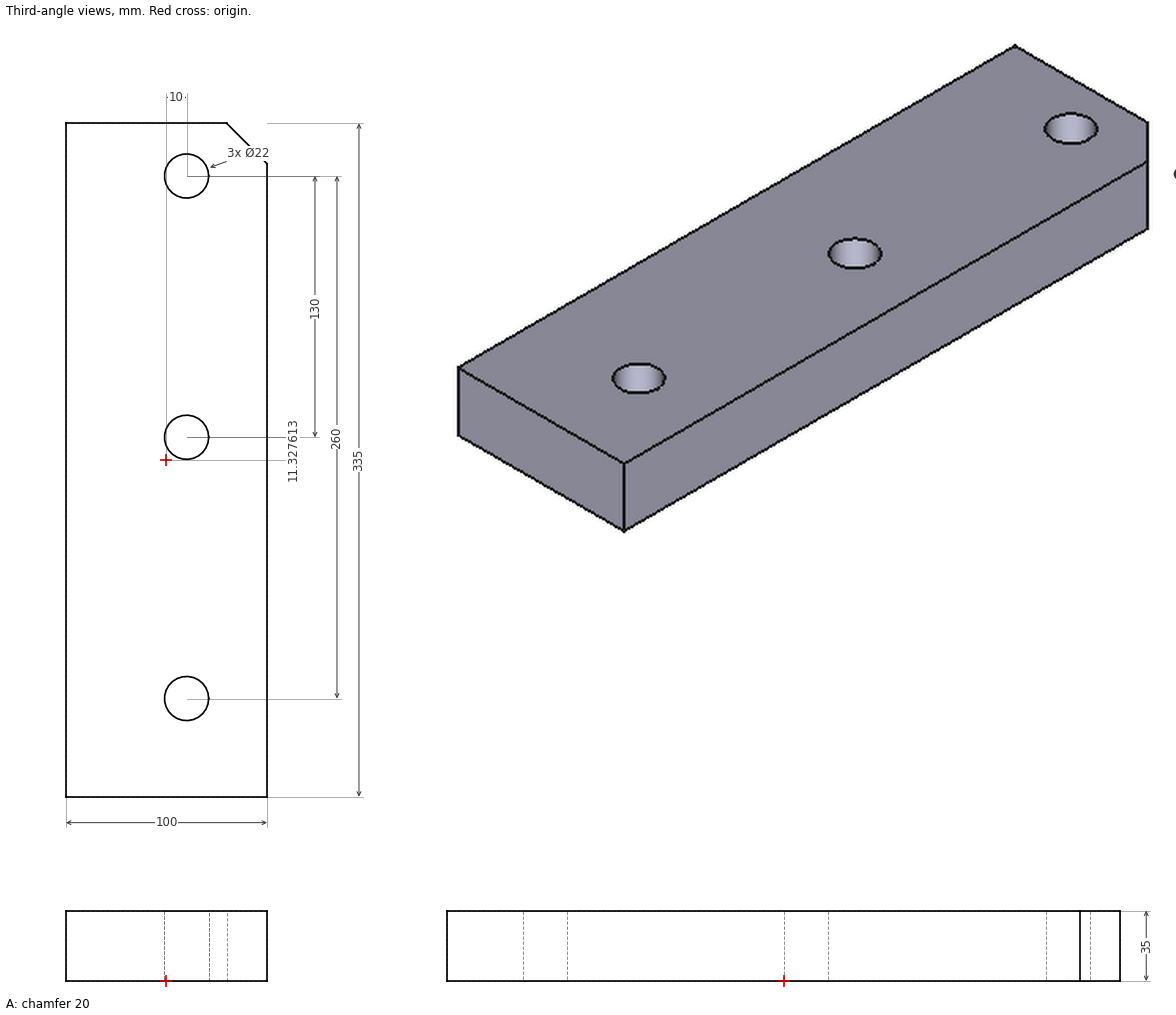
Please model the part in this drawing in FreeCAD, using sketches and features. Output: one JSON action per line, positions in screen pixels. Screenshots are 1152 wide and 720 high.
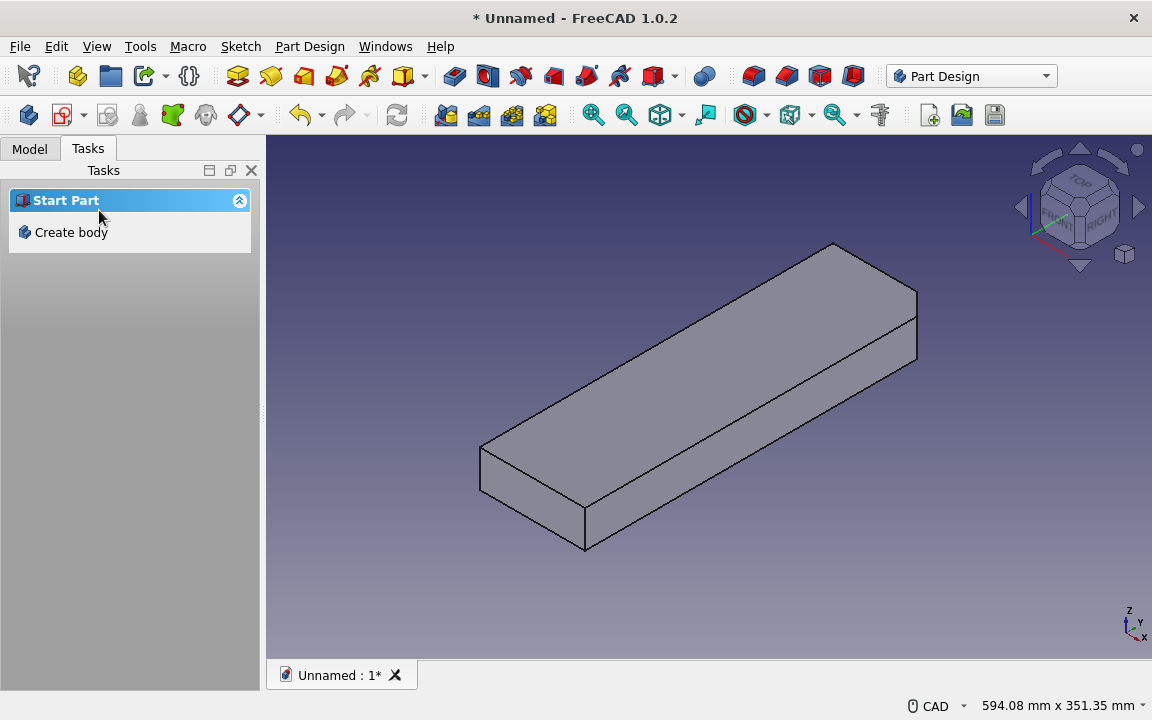
{"action": "left_click", "coordinate": [810, 316]}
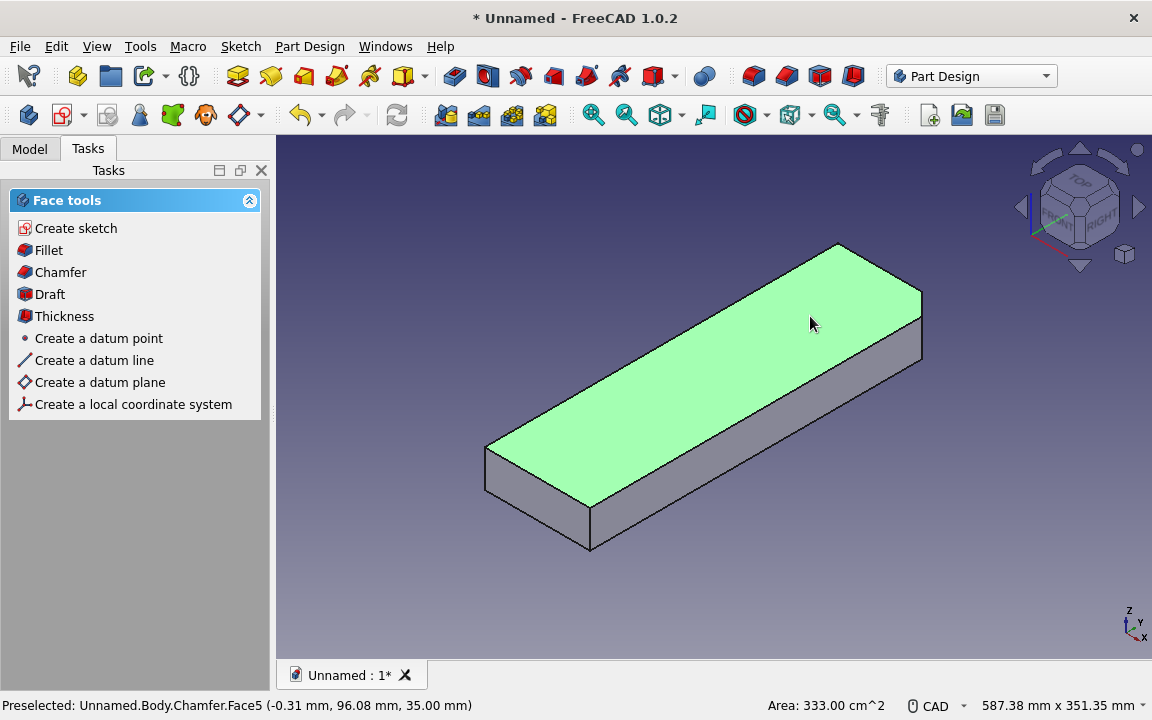
{"action": "left_click", "coordinate": [62, 116]}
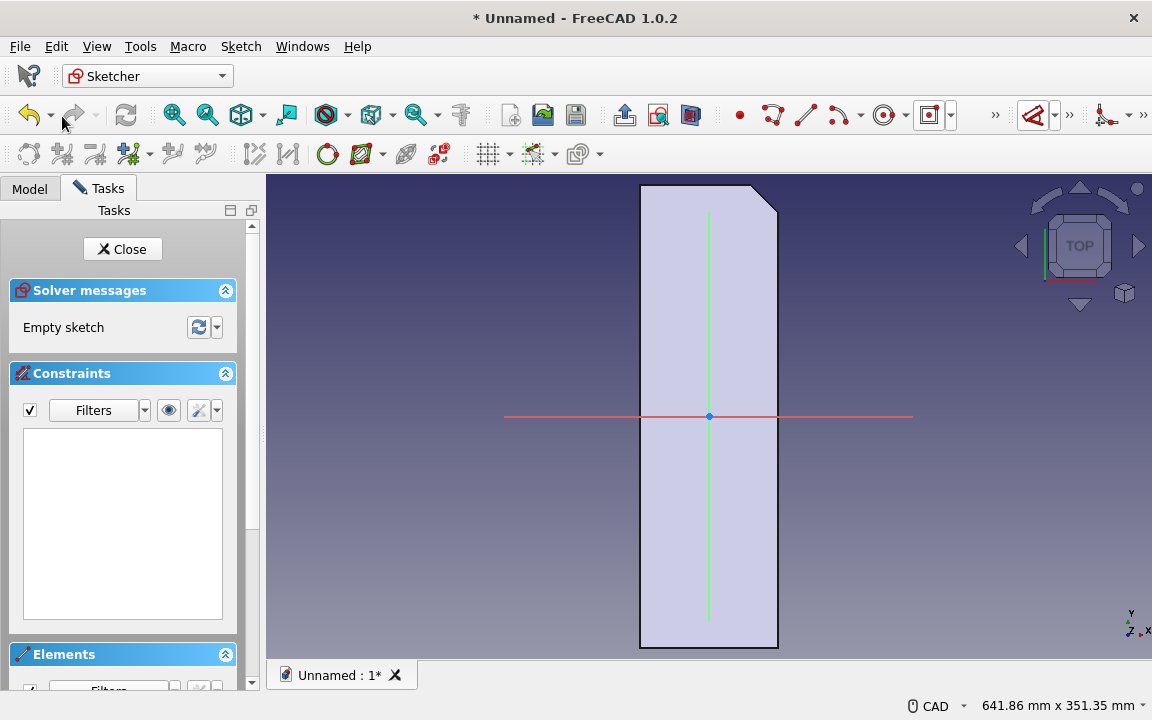
{"action": "scroll", "coordinate": [294, 487], "scroll_direction": "down", "scroll_amount": 1}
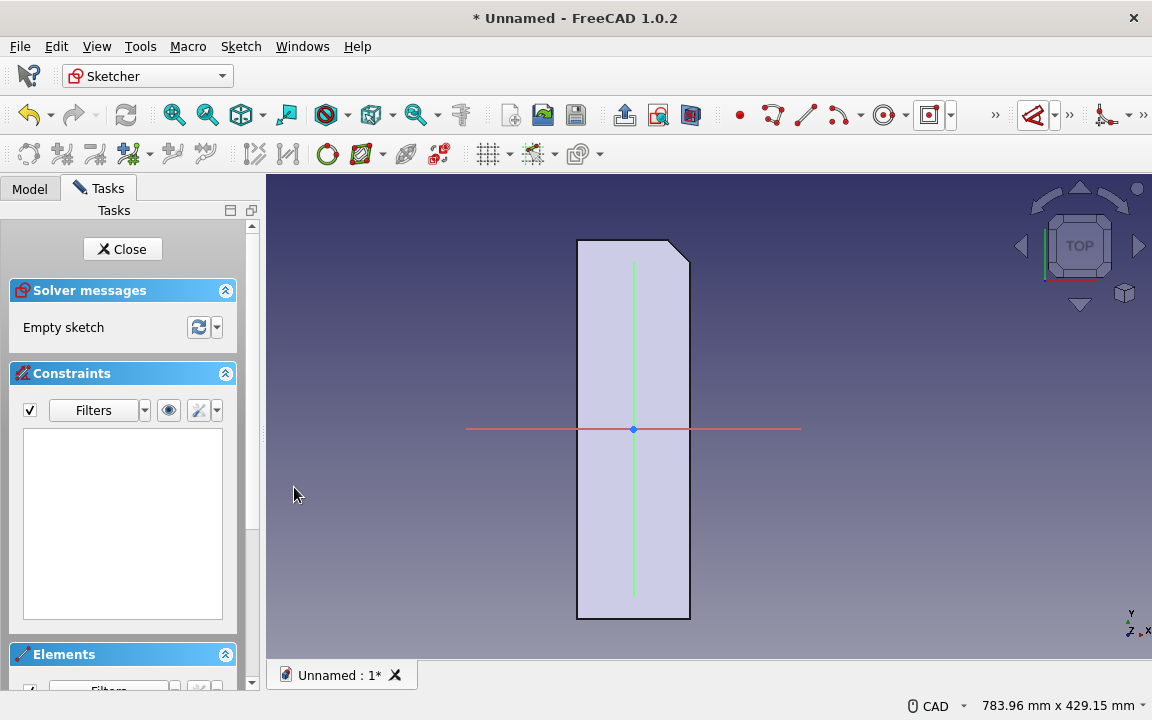
{"action": "left_click", "coordinate": [884, 116]}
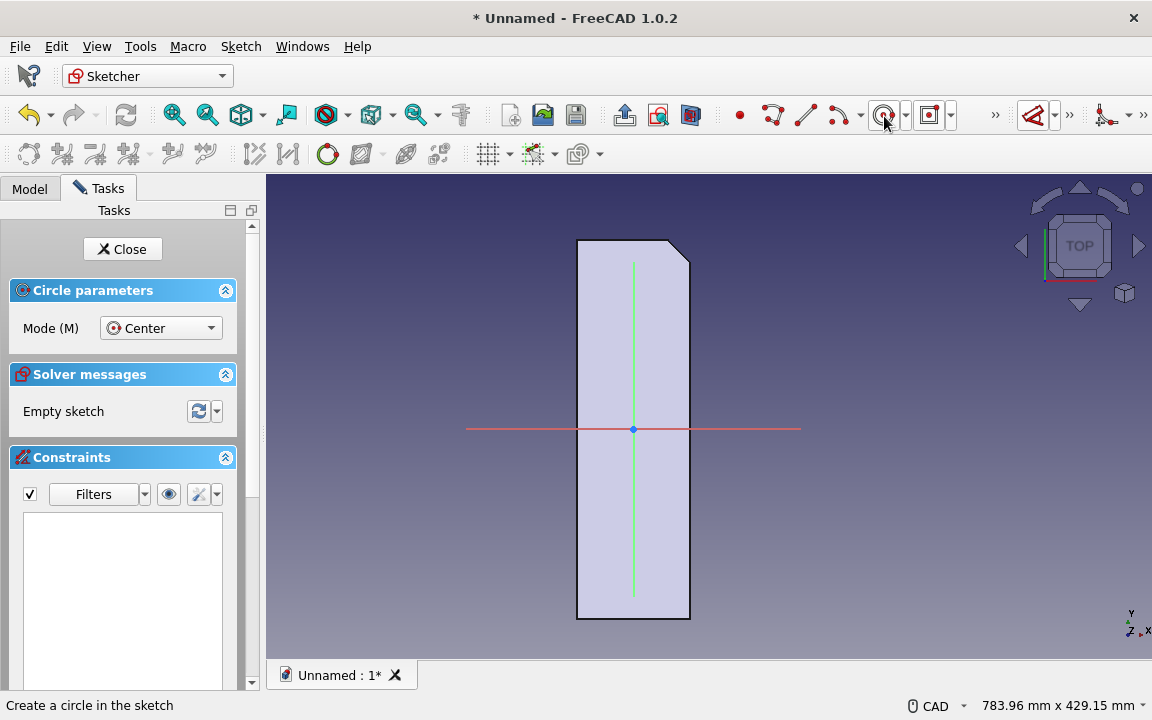
{"action": "scroll", "coordinate": [645, 270], "scroll_direction": "up", "scroll_amount": 4}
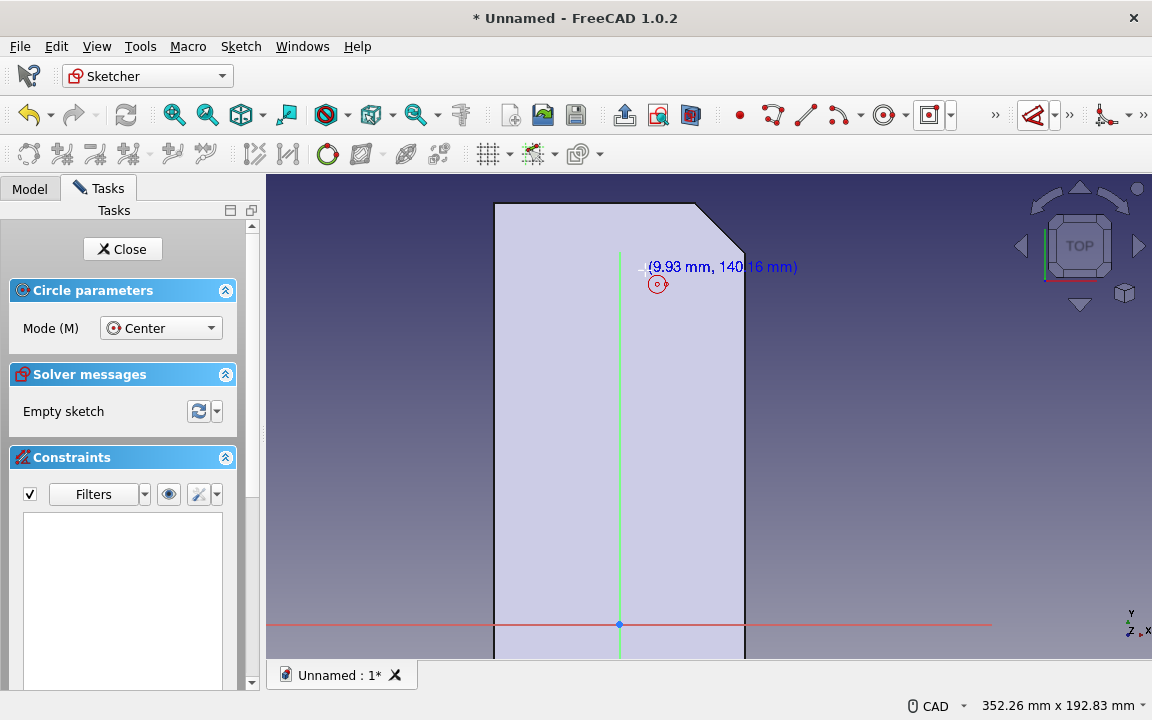
{"action": "left_click", "coordinate": [645, 269]}
{"action": "mouse_move", "coordinate": [664, 249]}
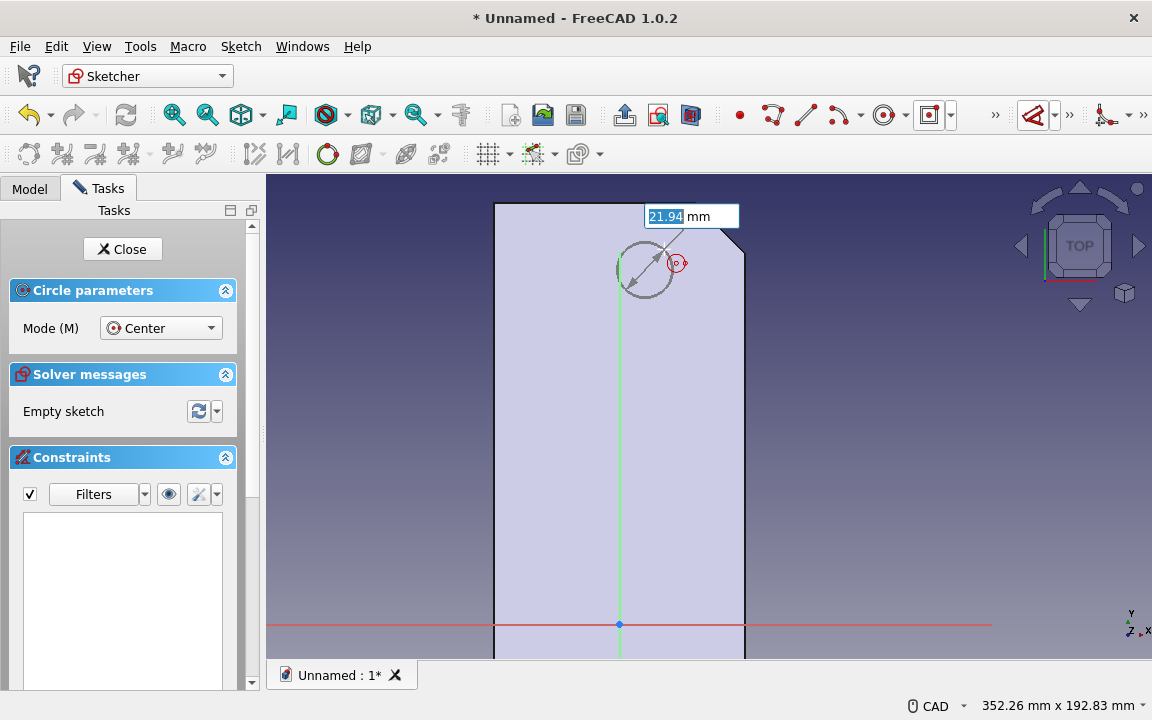
{"action": "type", "text": "22"}
{"action": "key", "text": "Return"}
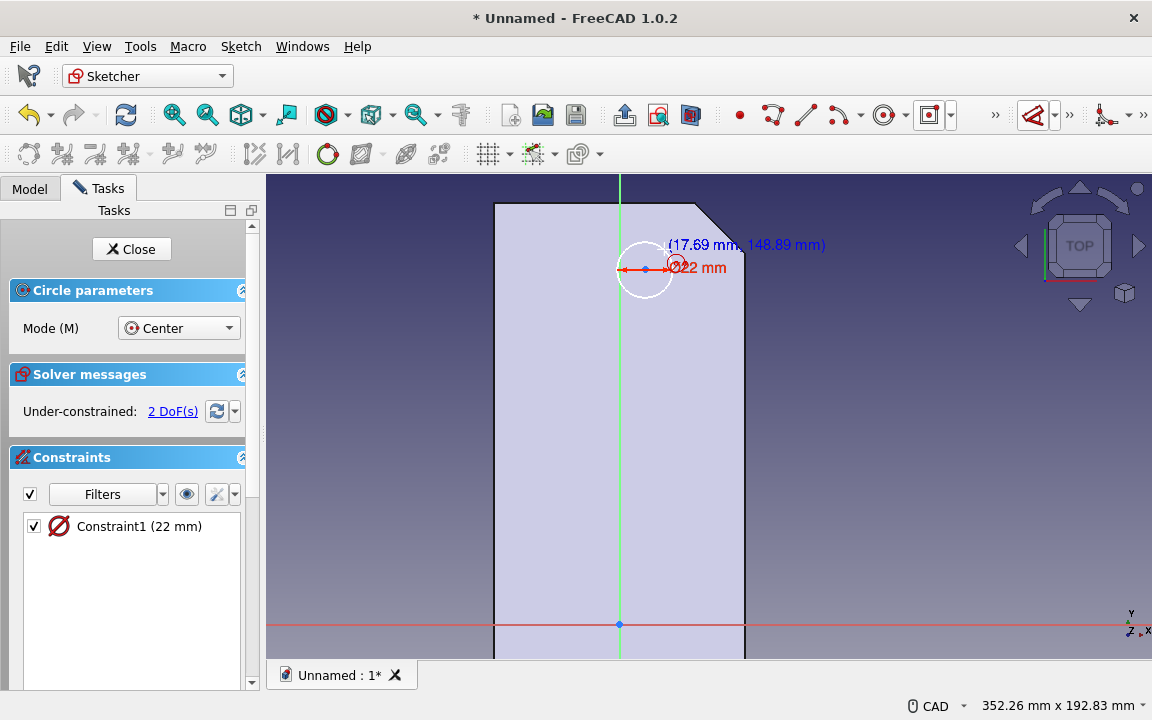
{"action": "scroll", "coordinate": [637, 270], "scroll_direction": "down", "scroll_amount": 4}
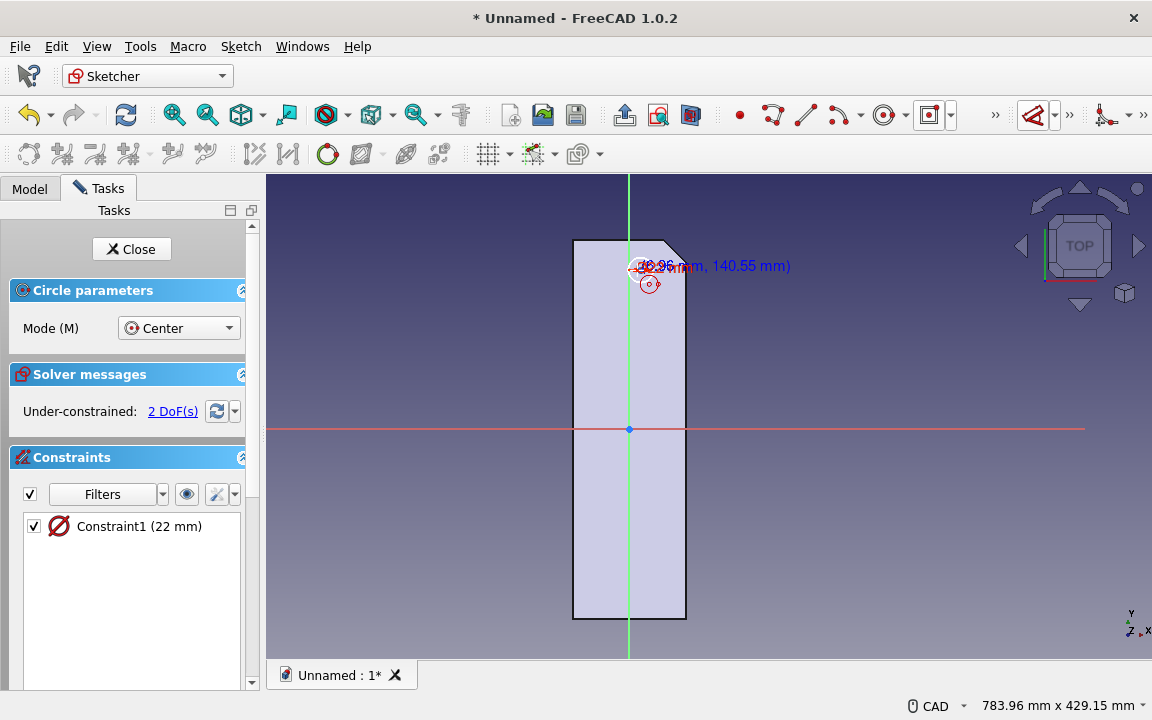
{"action": "scroll", "coordinate": [641, 564], "scroll_direction": "up", "scroll_amount": 4}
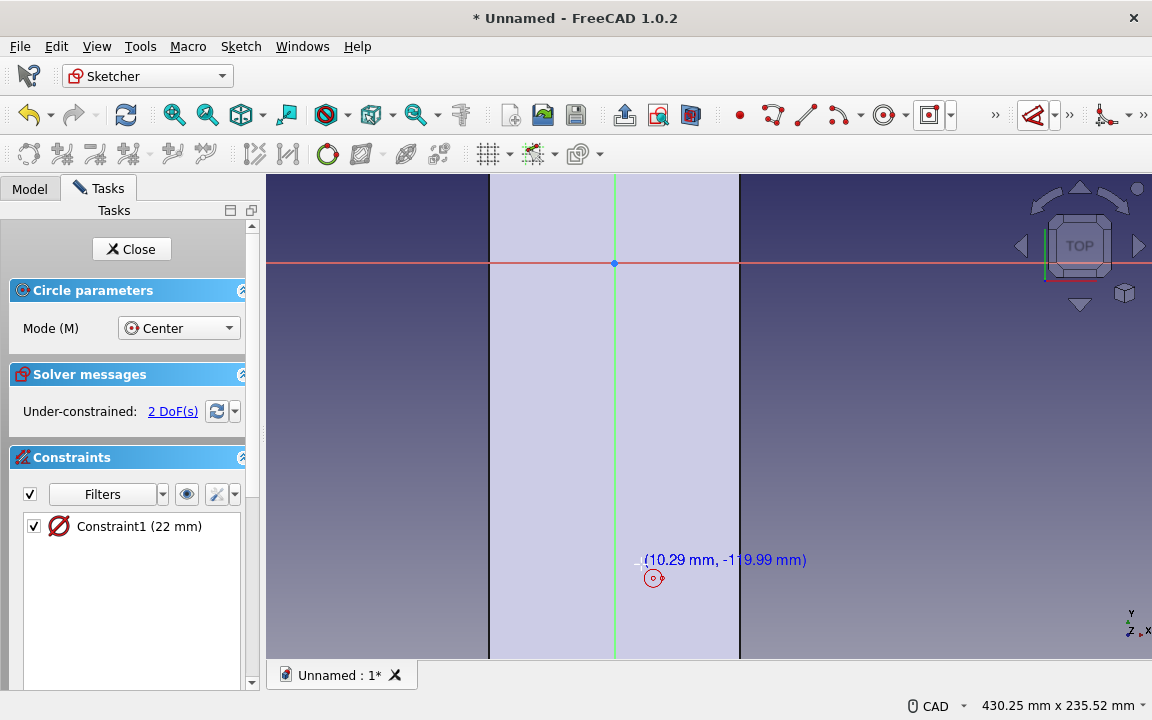
{"action": "left_click", "coordinate": [640, 562]}
{"action": "mouse_move", "coordinate": [659, 542]}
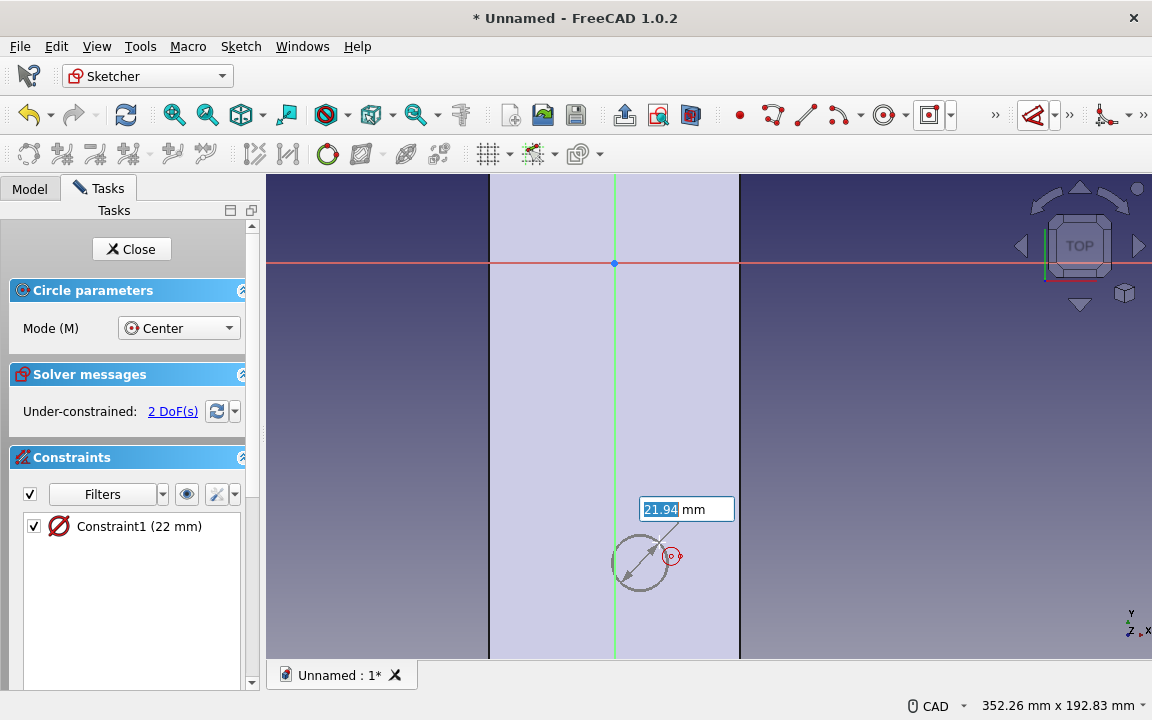
{"action": "type", "text": "22"}
{"action": "key", "text": "Return"}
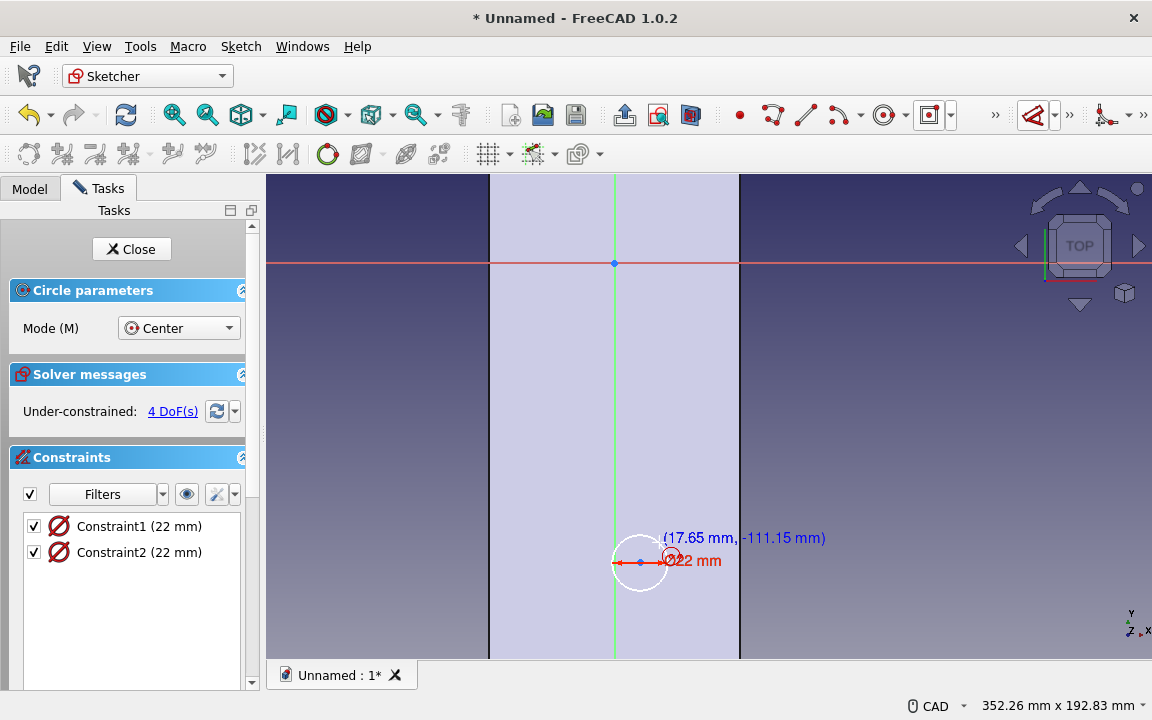
{"action": "left_click", "coordinate": [640, 235]}
{"action": "mouse_move", "coordinate": [659, 215]}